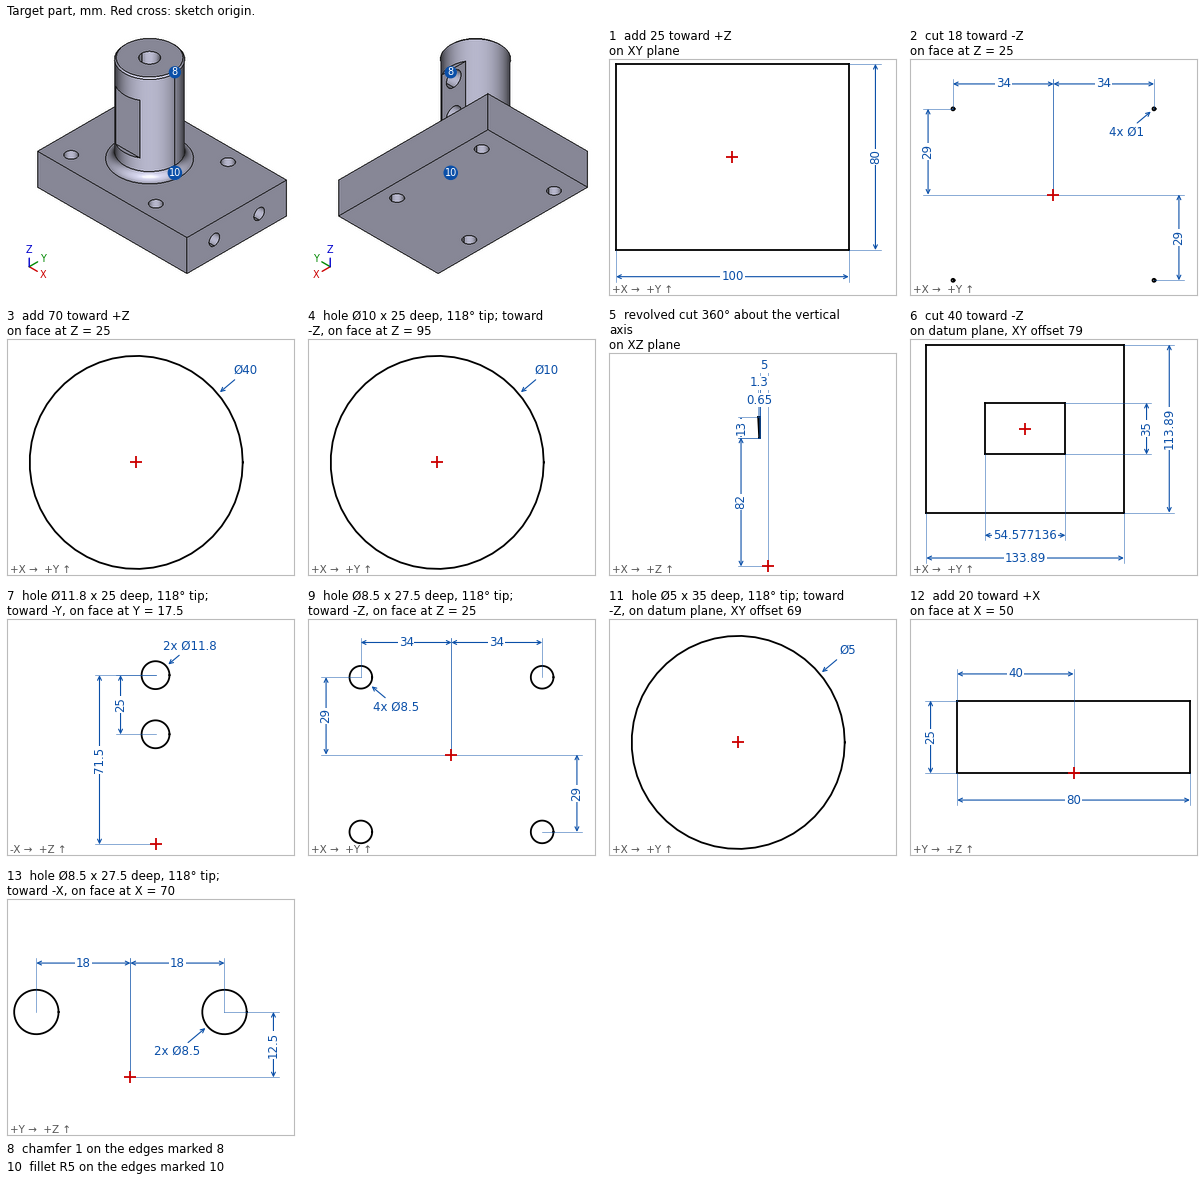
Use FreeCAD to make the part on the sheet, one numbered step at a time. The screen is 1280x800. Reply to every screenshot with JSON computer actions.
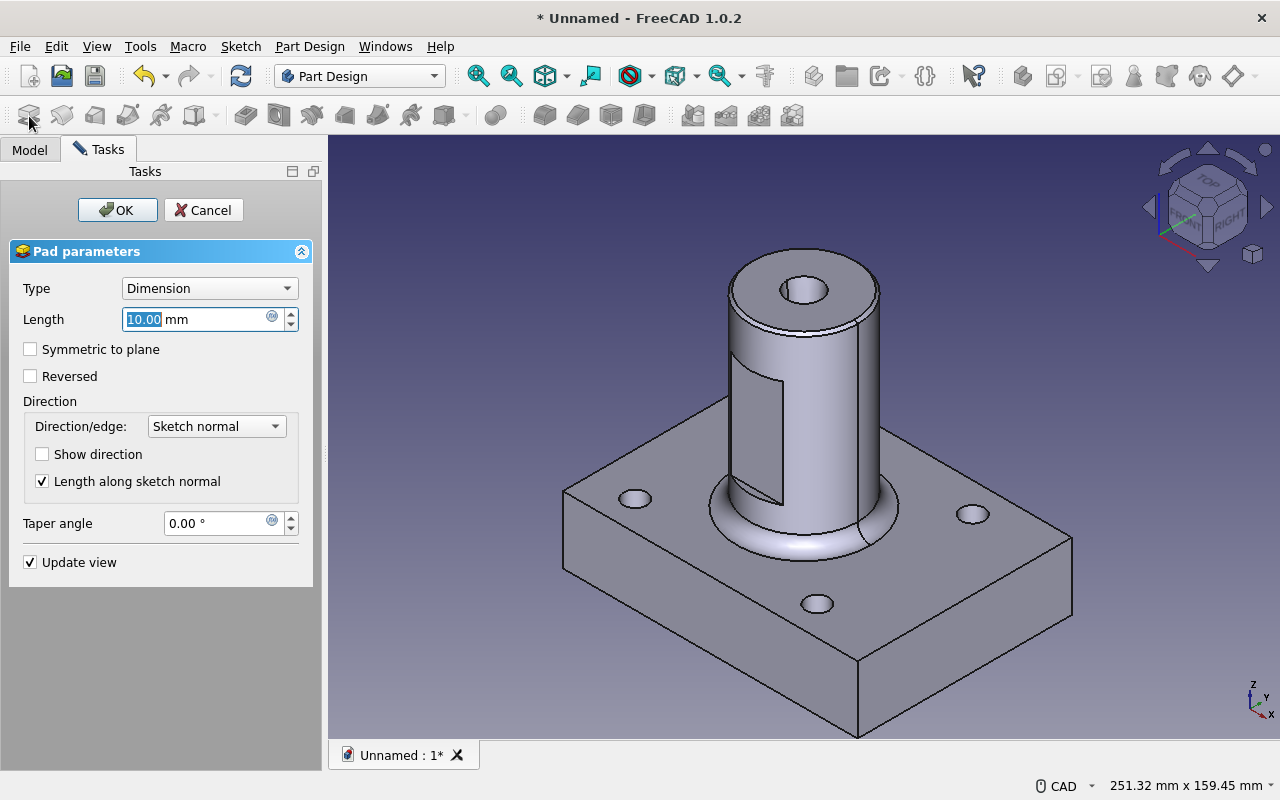
{"action": "type", "text": "20"}
{"action": "key", "text": "Tab"}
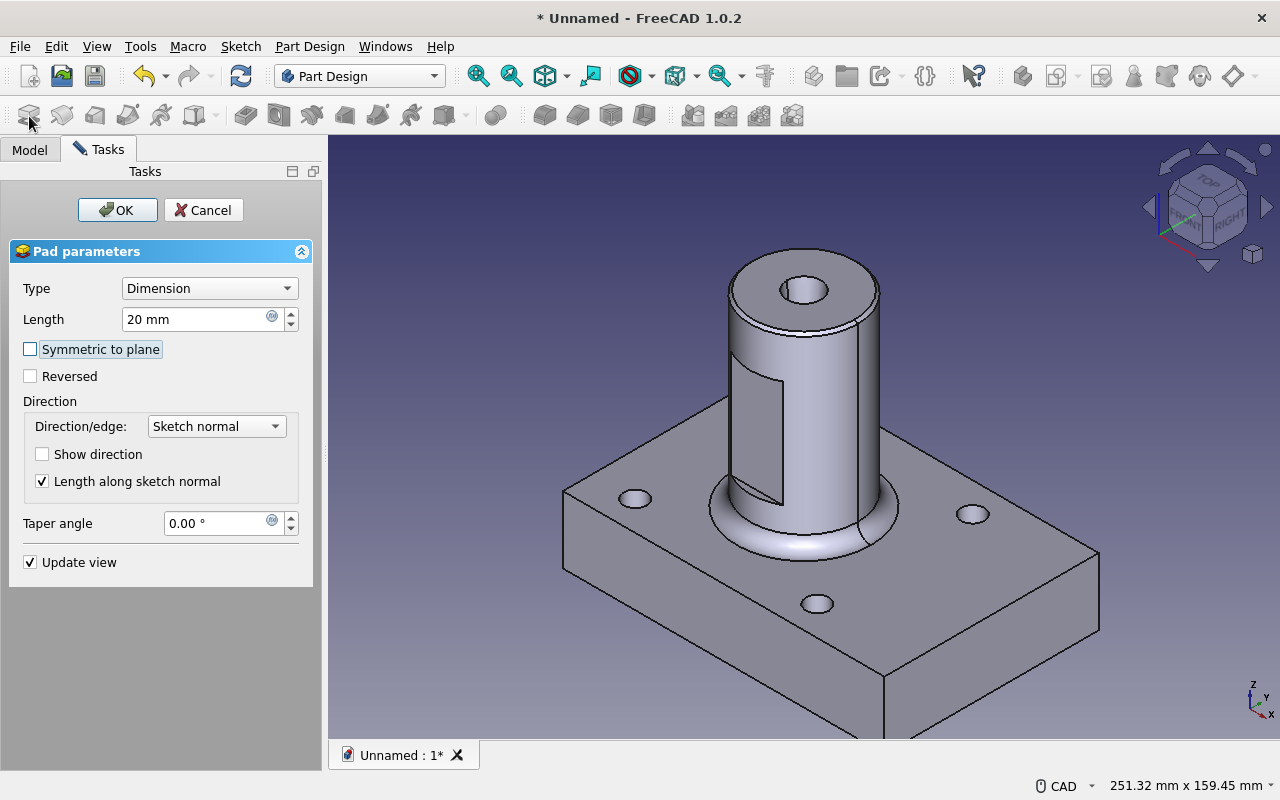
{"action": "left_click", "coordinate": [118, 210]}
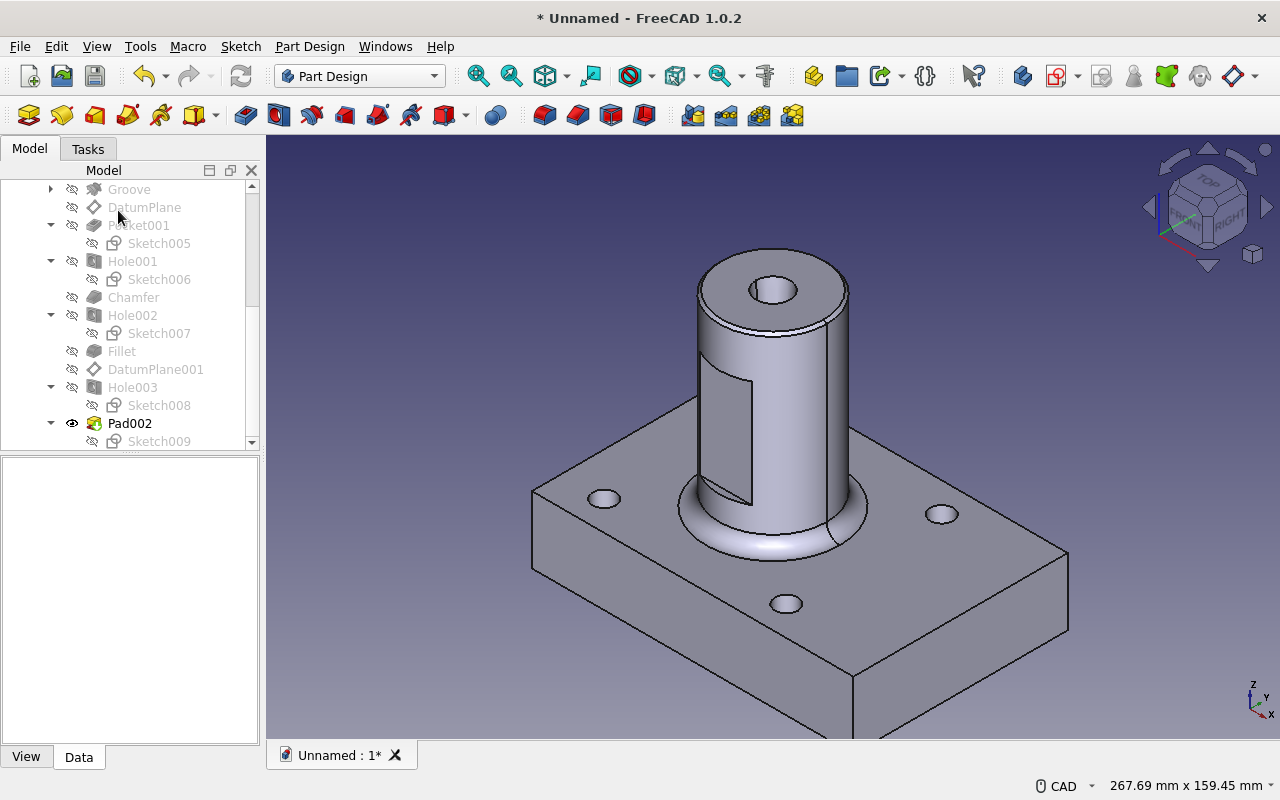
{"action": "left_click", "coordinate": [479, 76]}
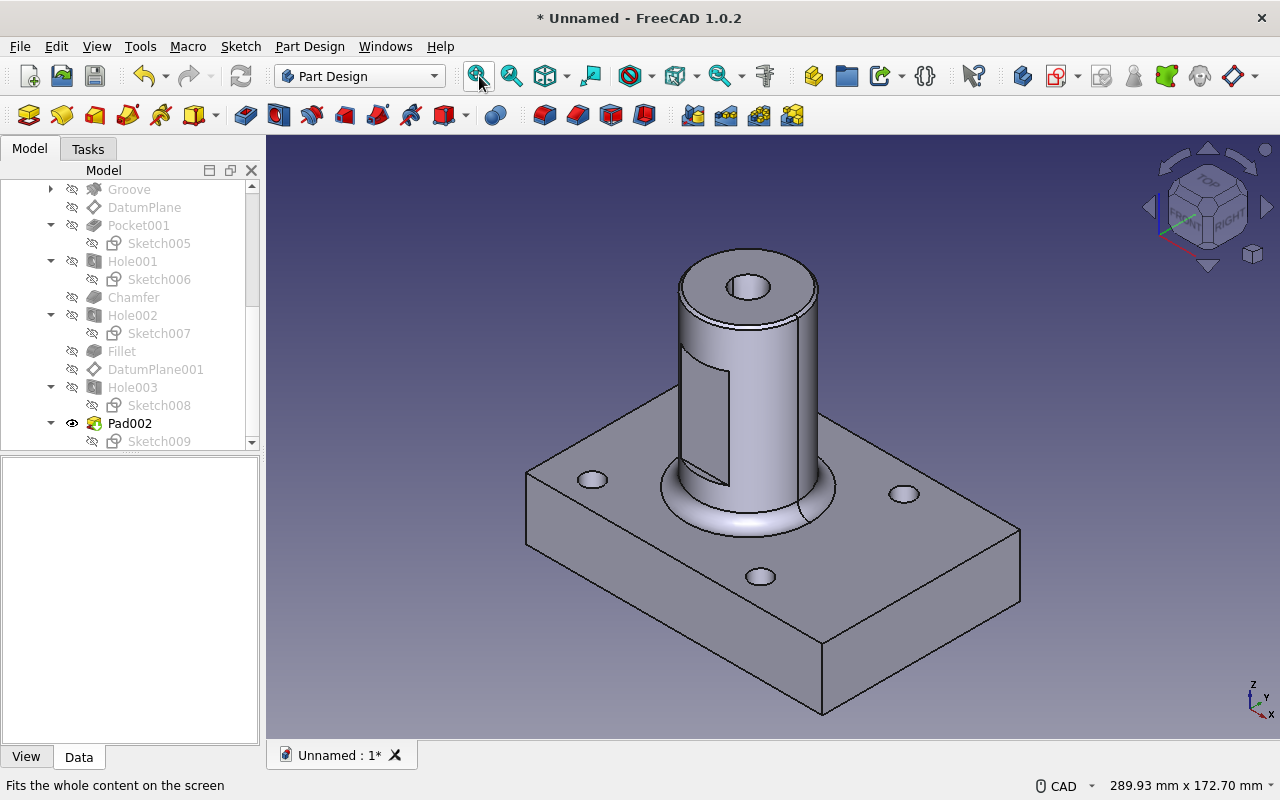
{"action": "left_click", "coordinate": [978, 589]}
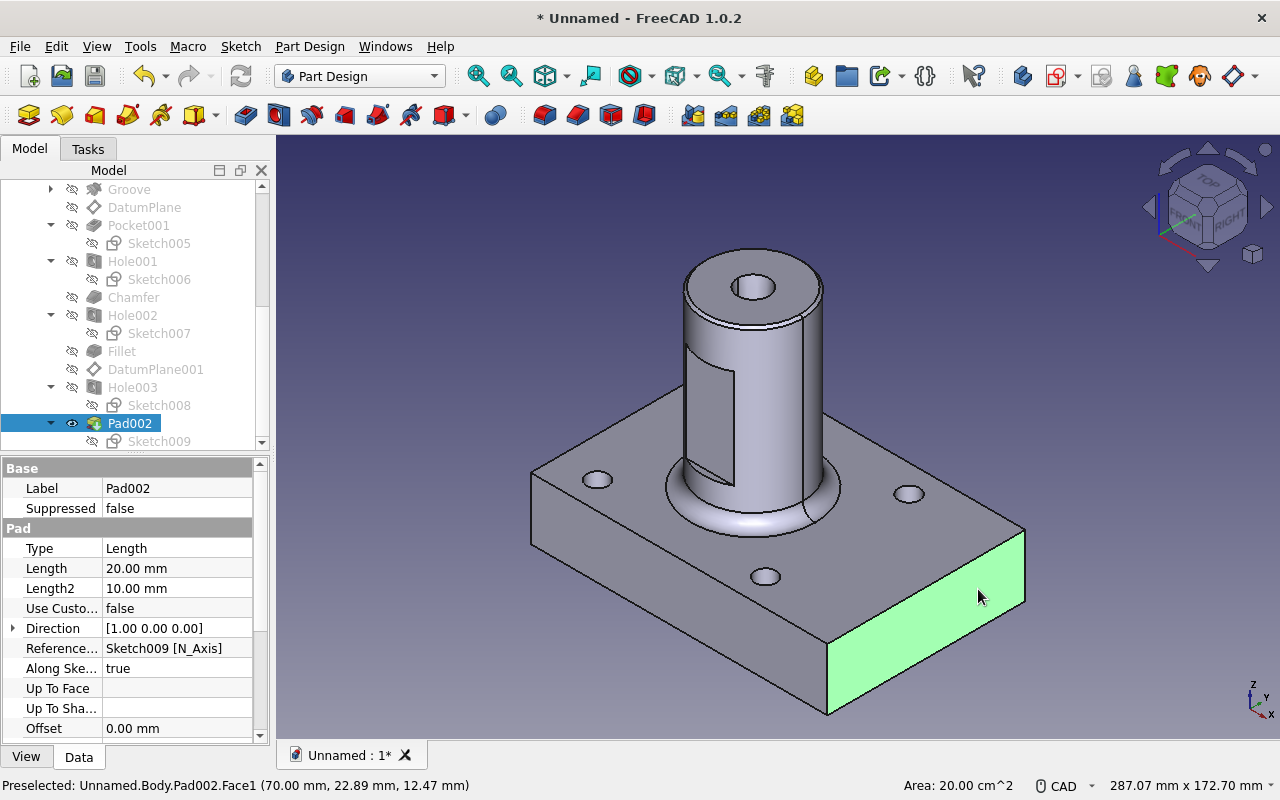
{"action": "left_click", "coordinate": [1056, 76]}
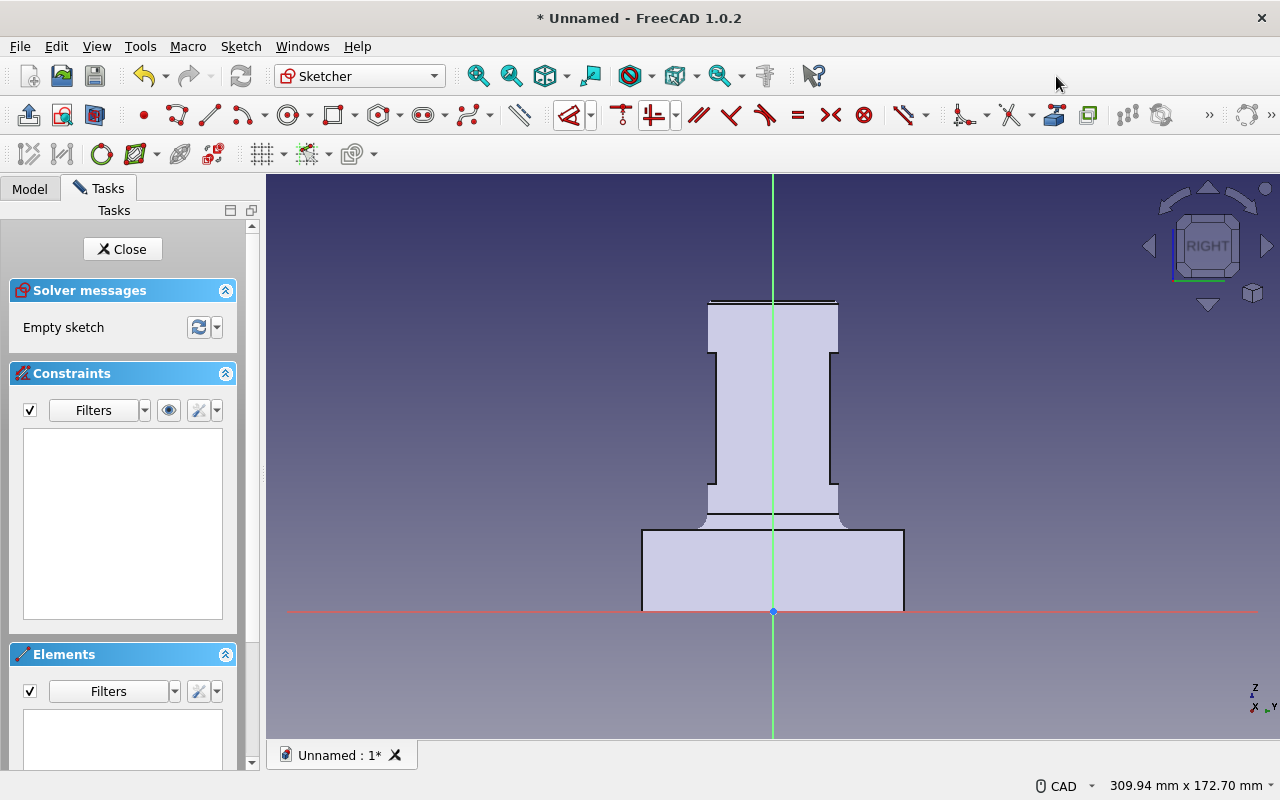
{"action": "scroll", "coordinate": [795, 626], "scroll_direction": "up", "scroll_amount": 7}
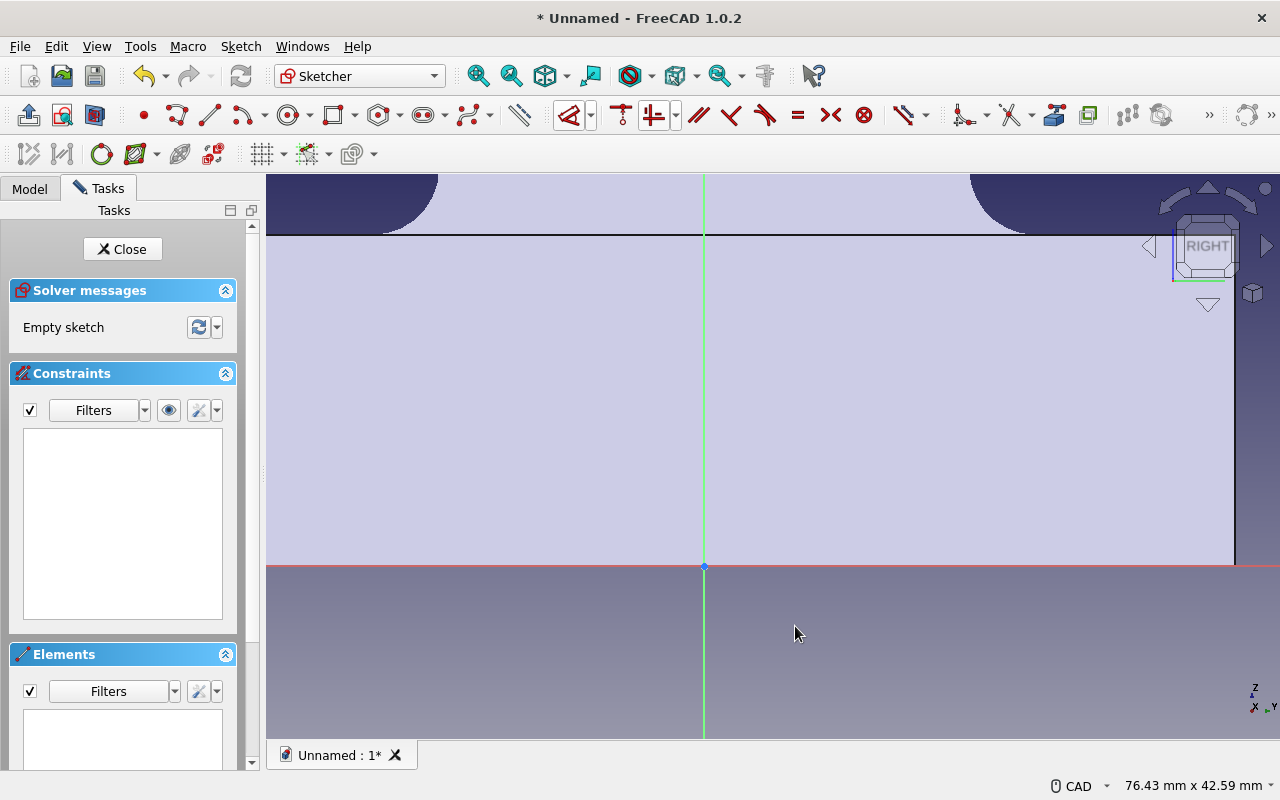
{"action": "key", "text": "g c"}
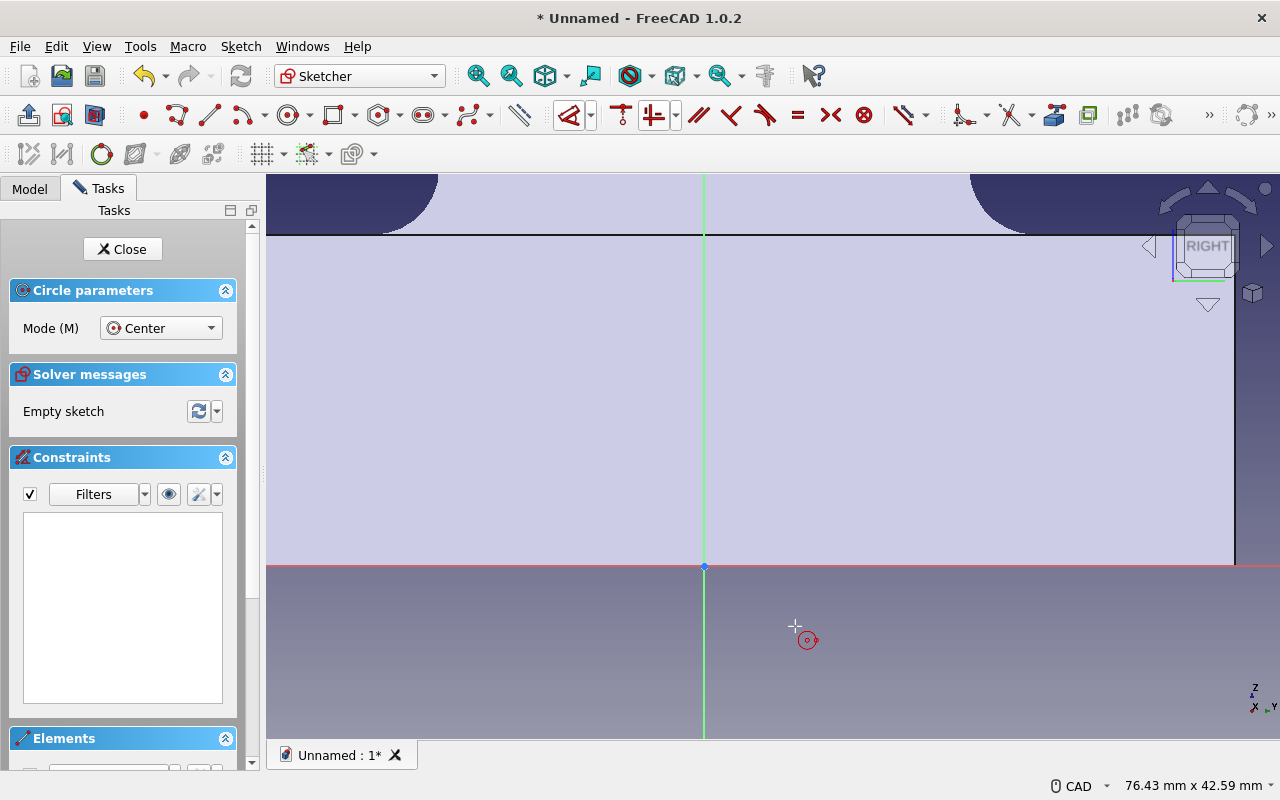
{"action": "left_click", "coordinate": [943, 401]}
{"action": "mouse_move", "coordinate": [983, 361]}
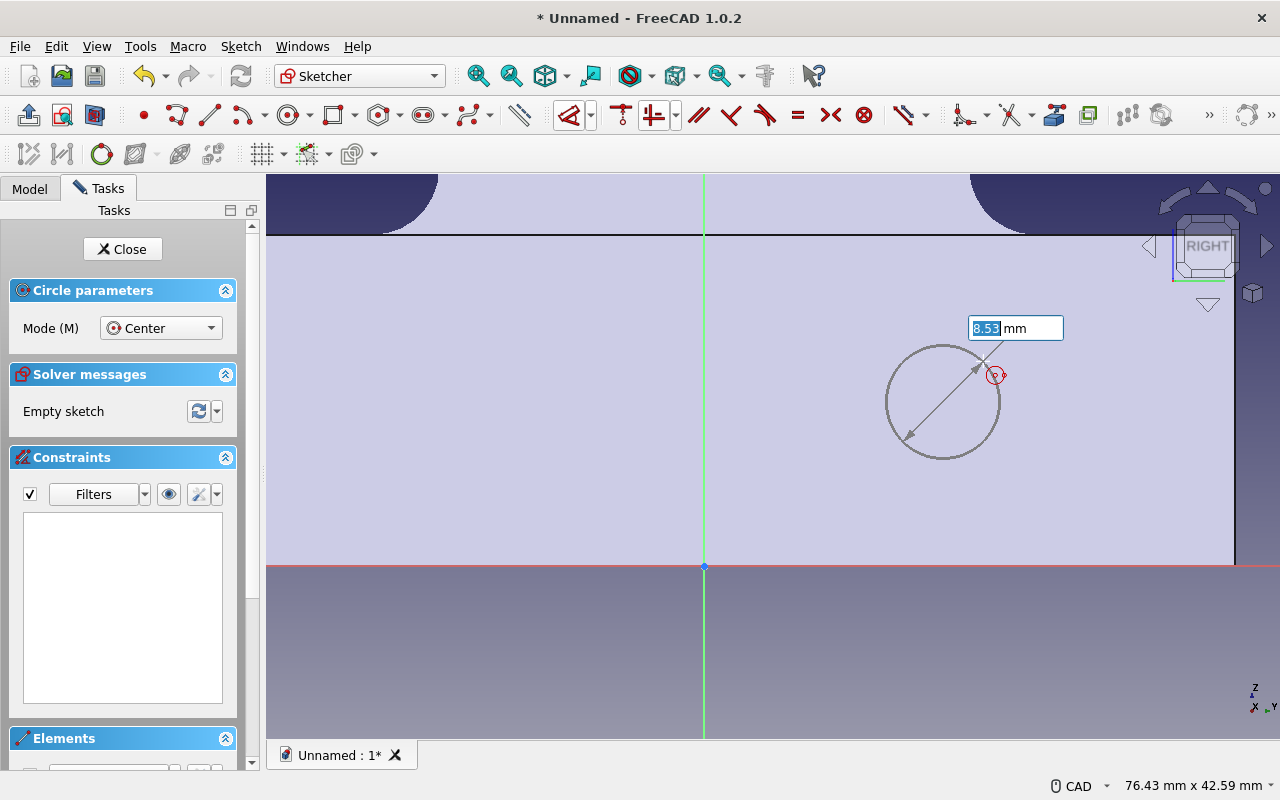
{"action": "type", "text": "8.5"}
{"action": "key", "text": "Return"}